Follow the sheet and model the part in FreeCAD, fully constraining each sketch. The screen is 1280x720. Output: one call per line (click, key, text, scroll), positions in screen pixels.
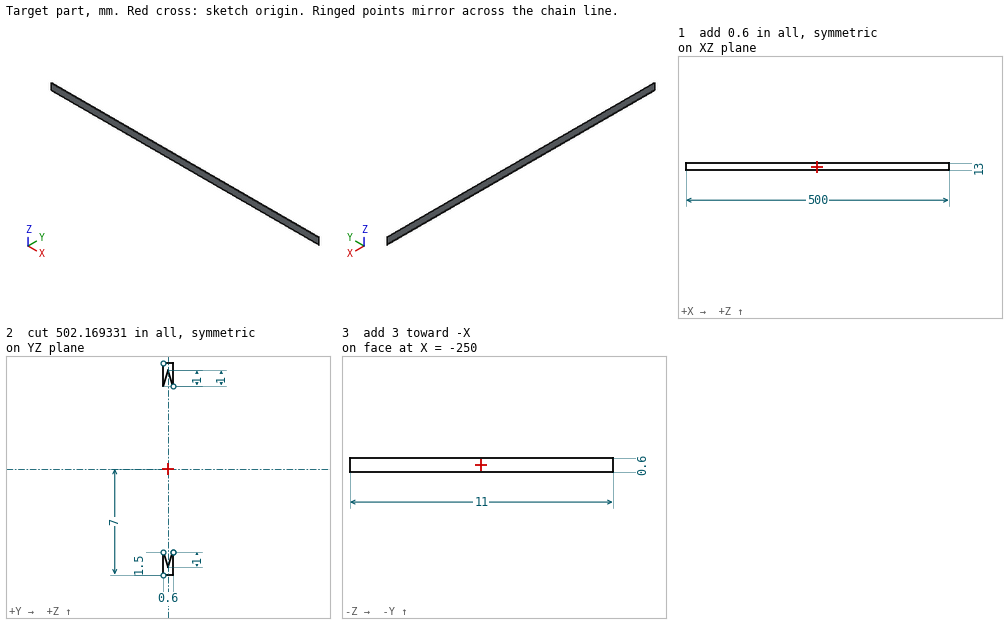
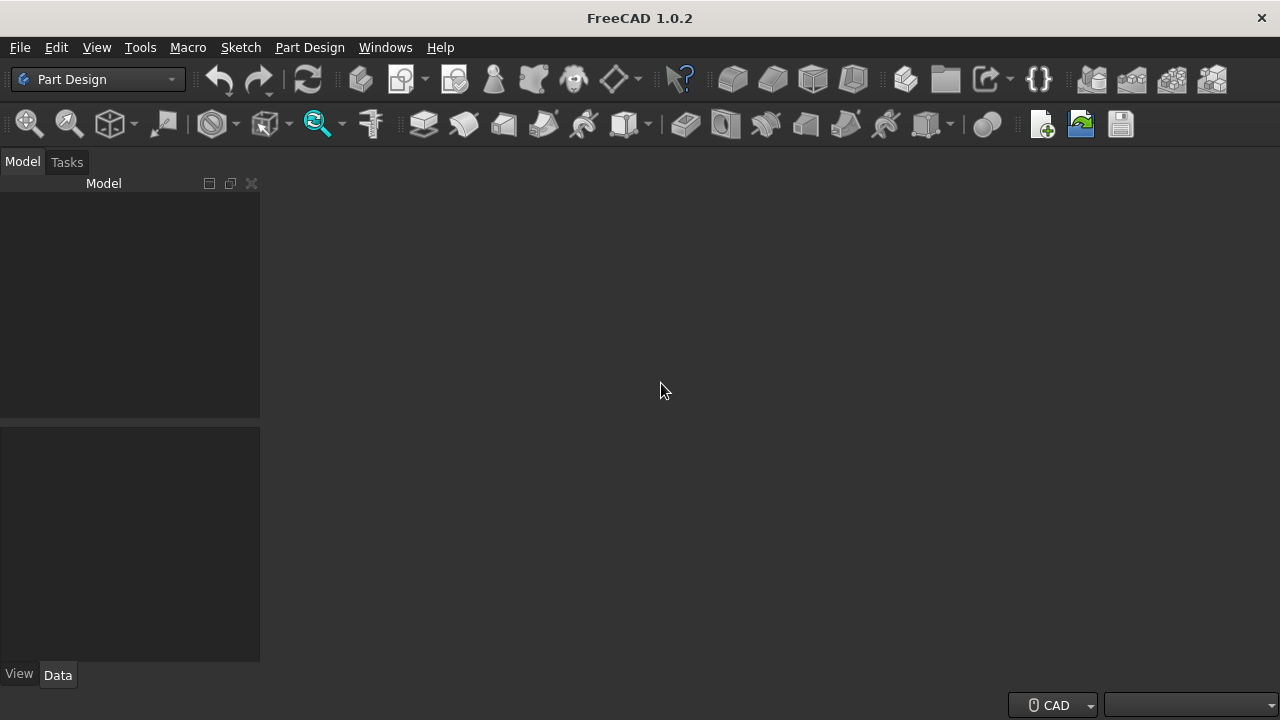
click(1042, 124)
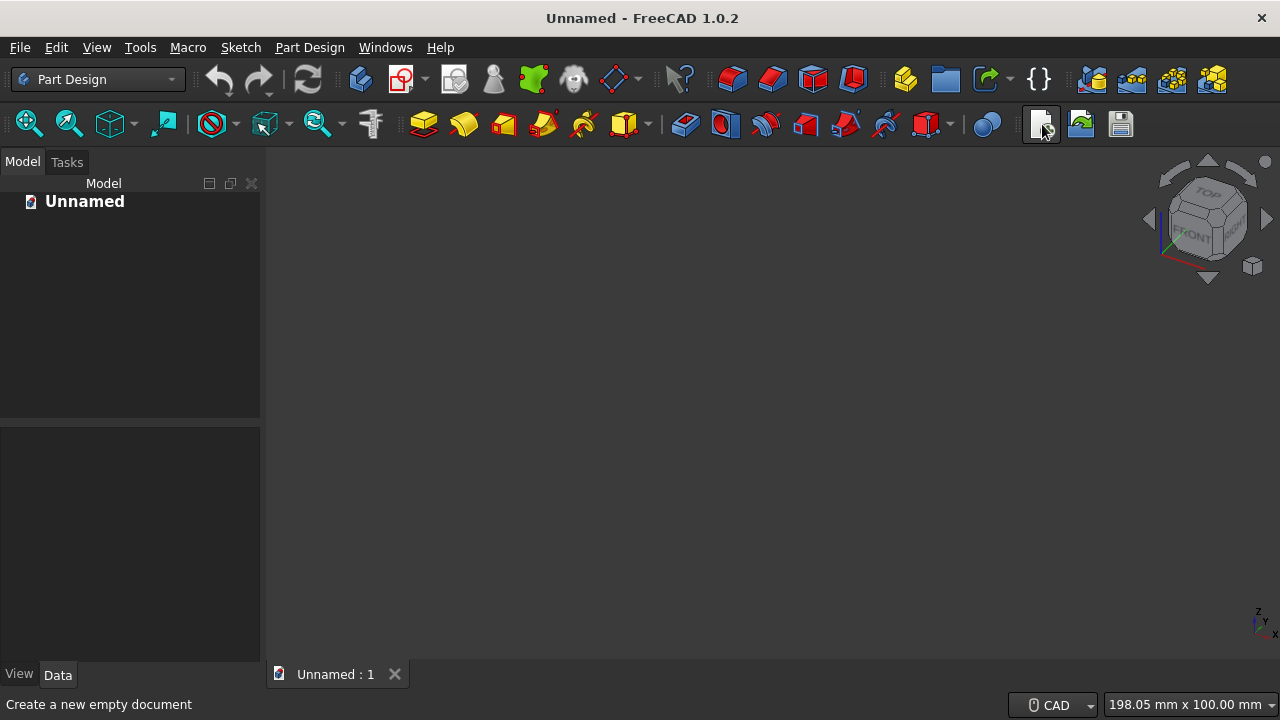
click(402, 80)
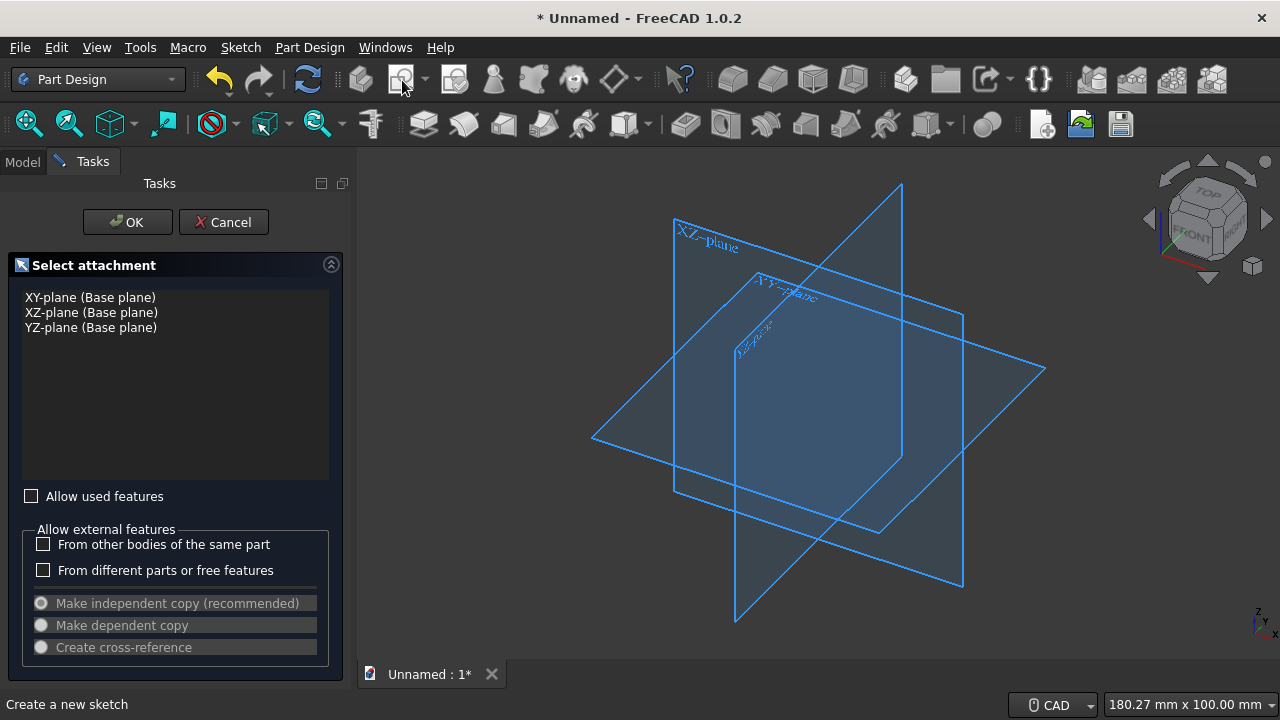
click(82, 312)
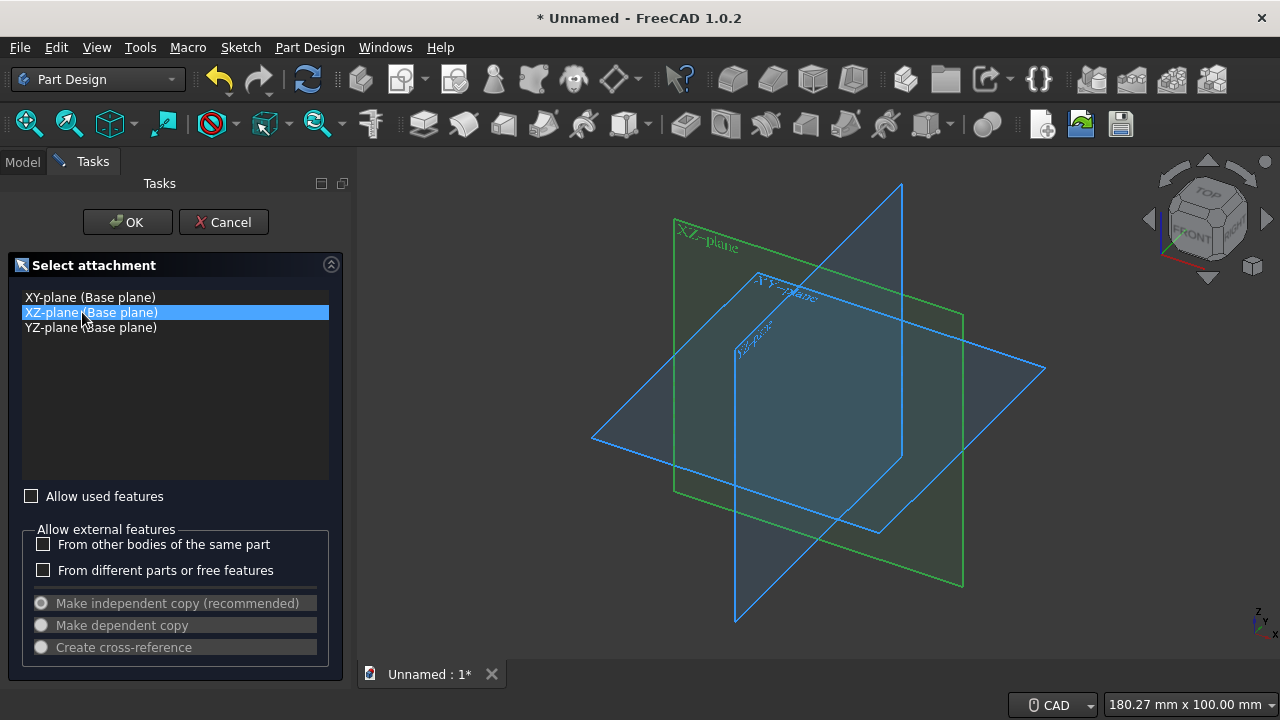
click(128, 222)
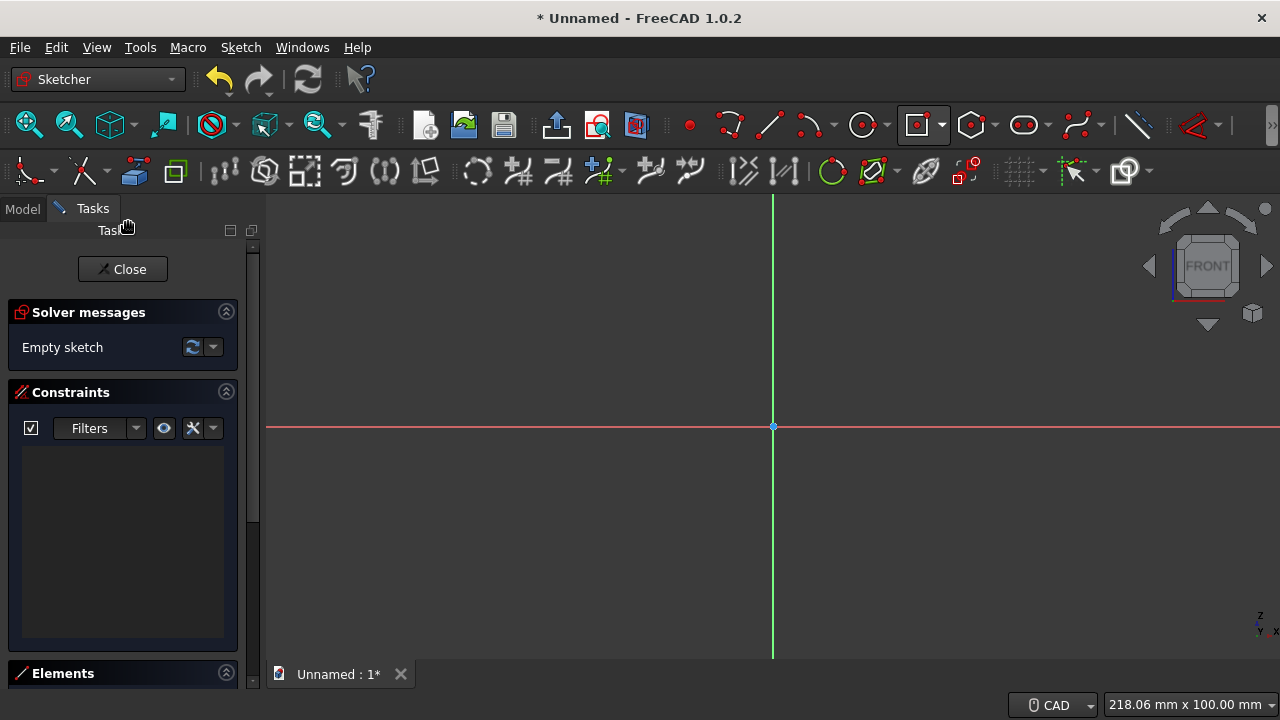
scroll(682, 426, down, 7)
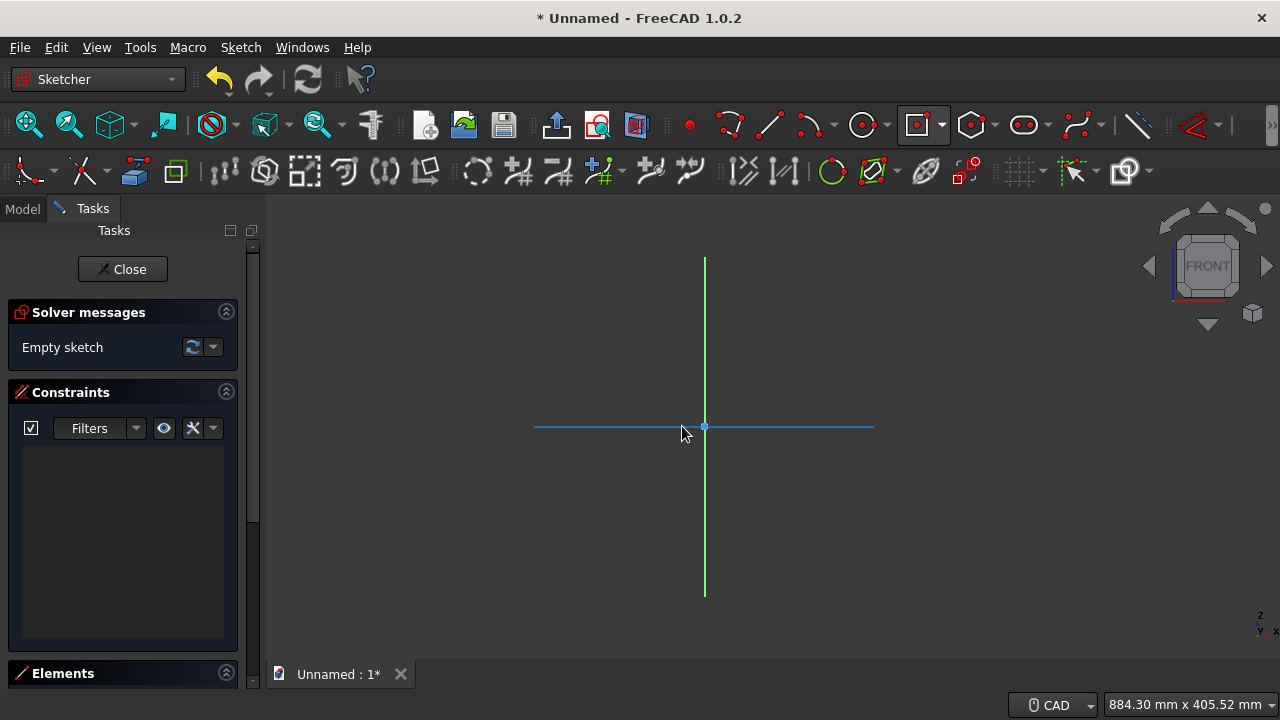
click(918, 126)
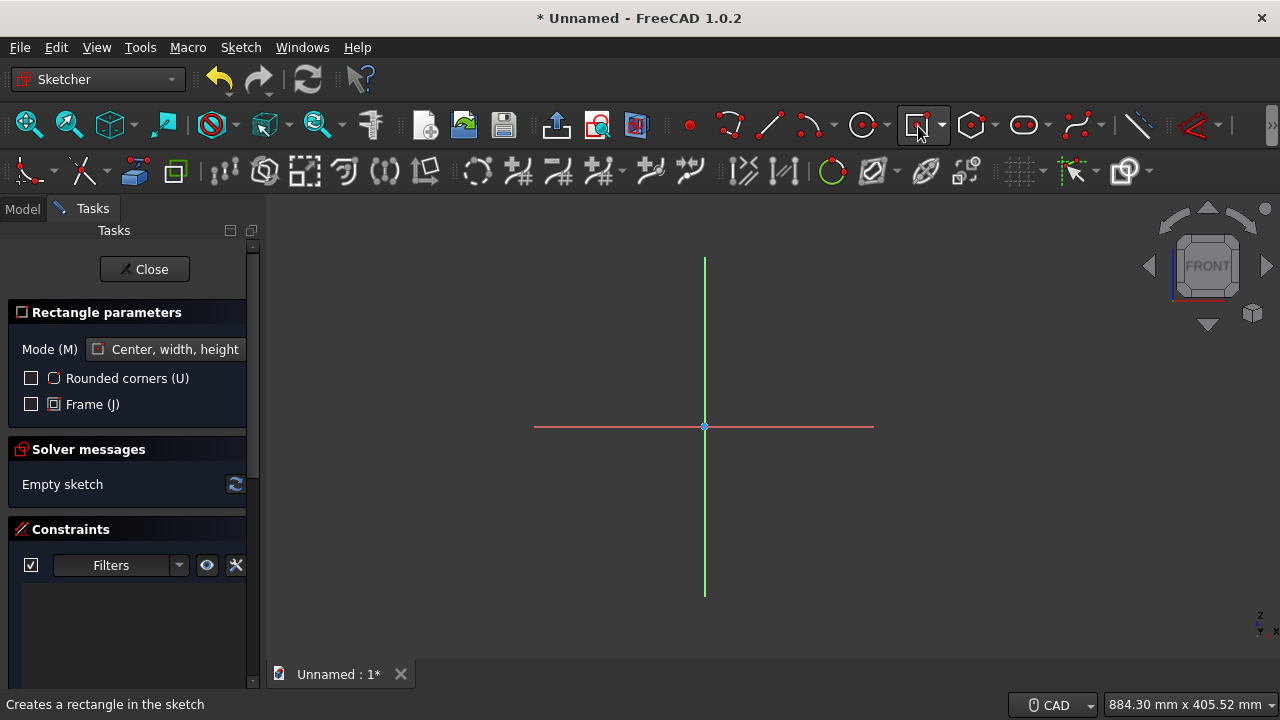
scroll(705, 426, up, 4)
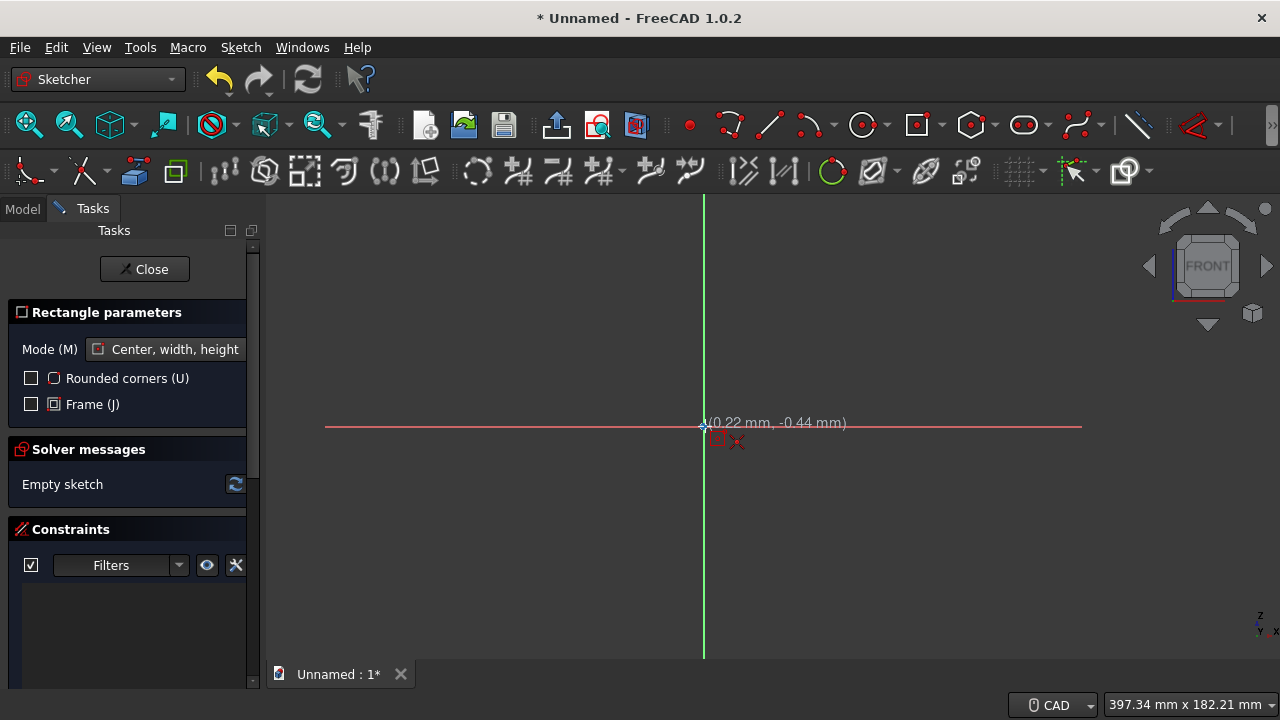
click(704, 426)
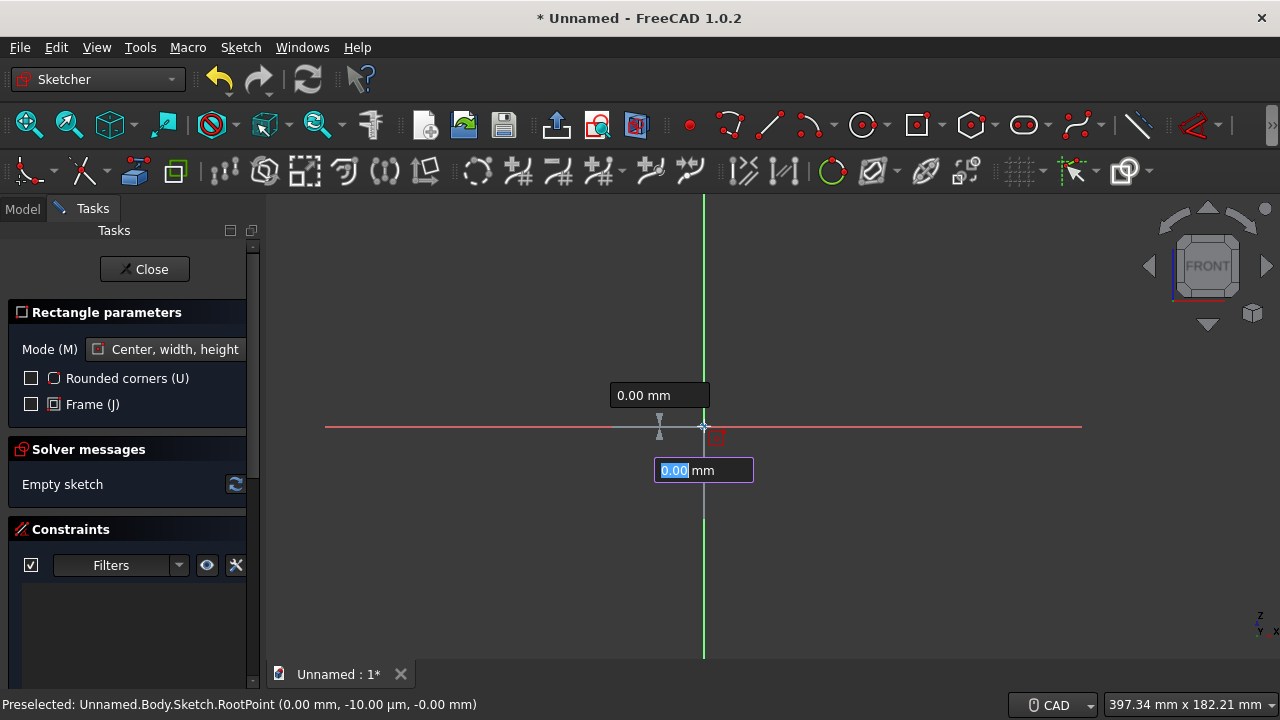
scroll(705, 426, down, 4)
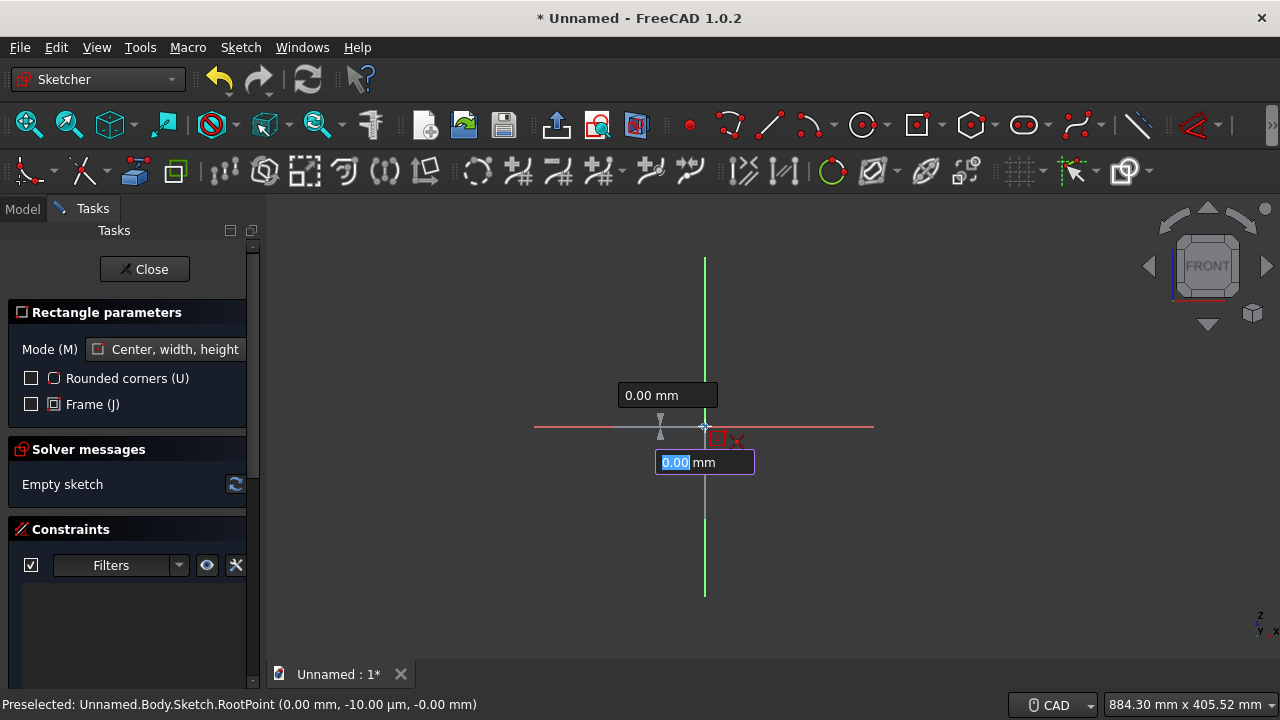
scroll(991, 419, up, 4)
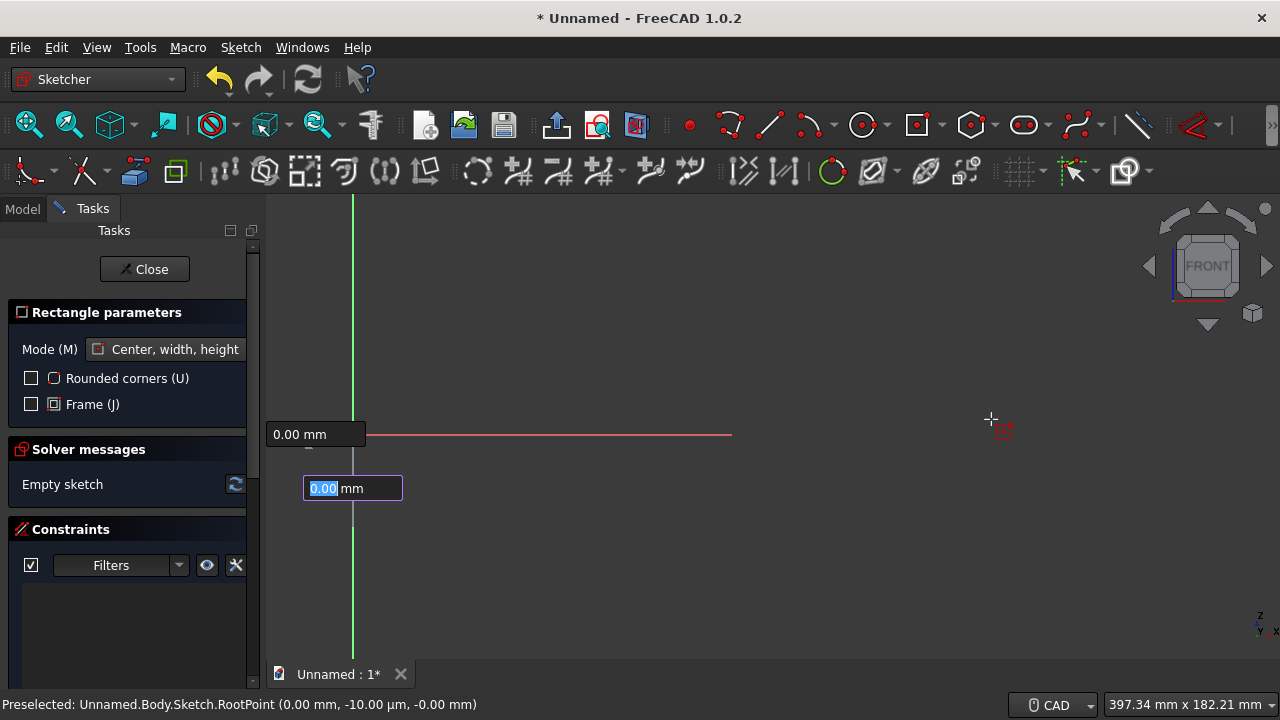
click(991, 419)
key(Escape)